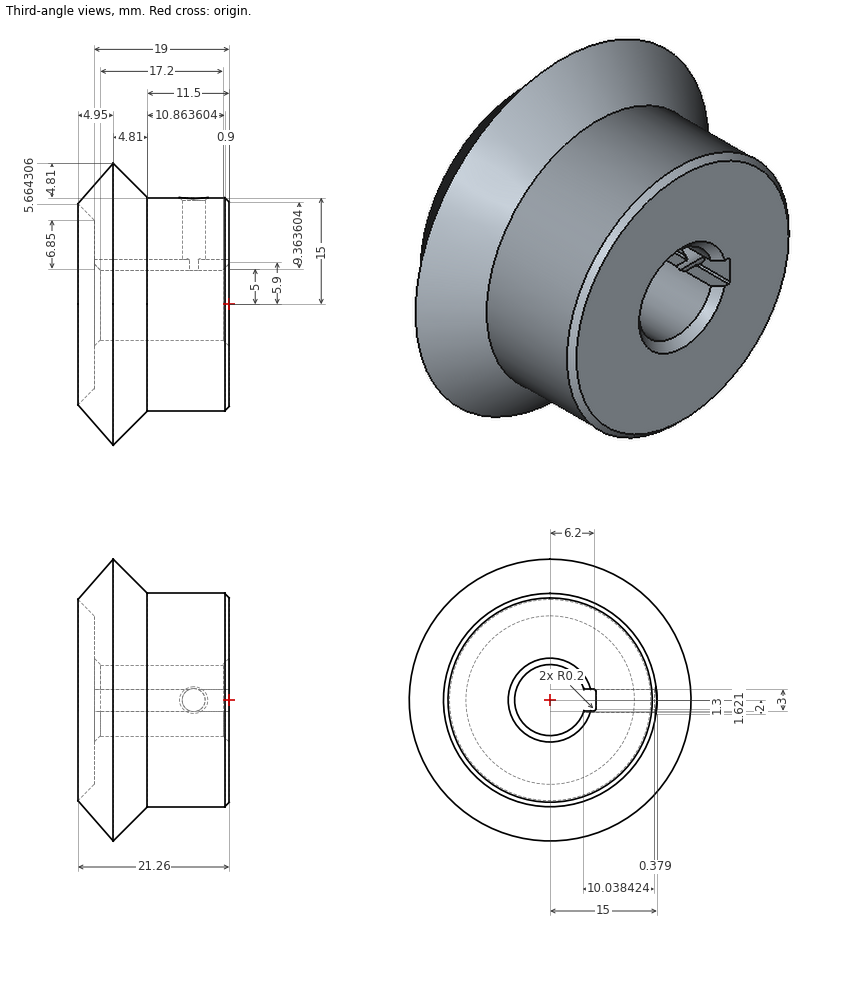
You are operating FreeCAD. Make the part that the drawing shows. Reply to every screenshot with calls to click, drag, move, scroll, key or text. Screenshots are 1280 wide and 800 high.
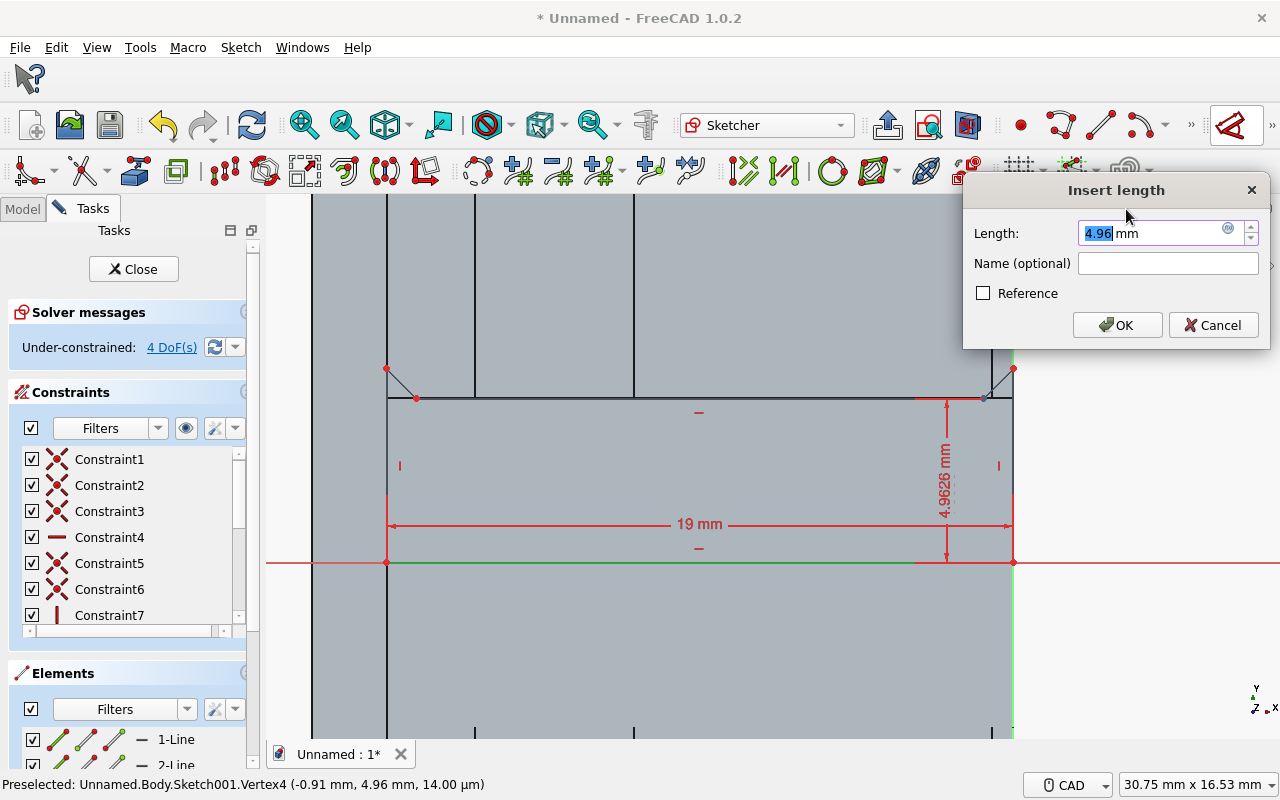
text(5)
key(Return)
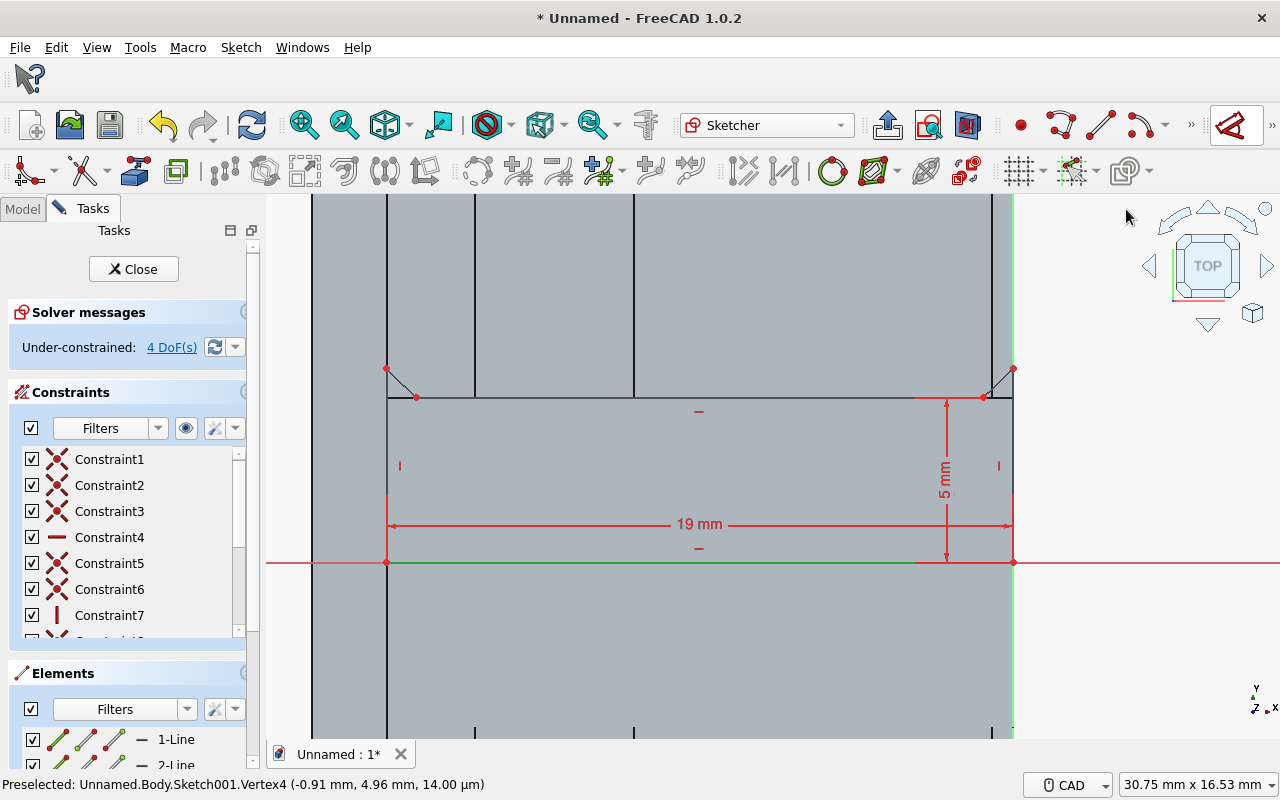
click(1013, 505)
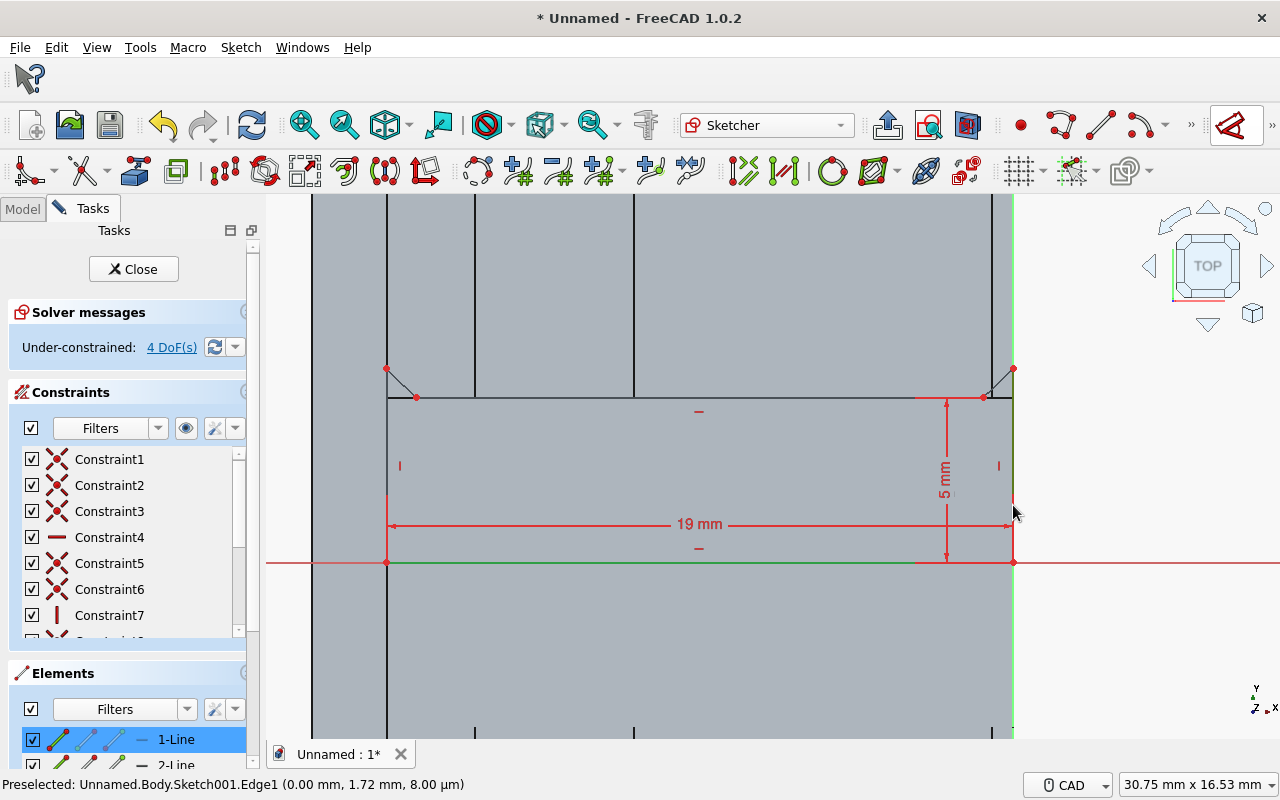
key(i)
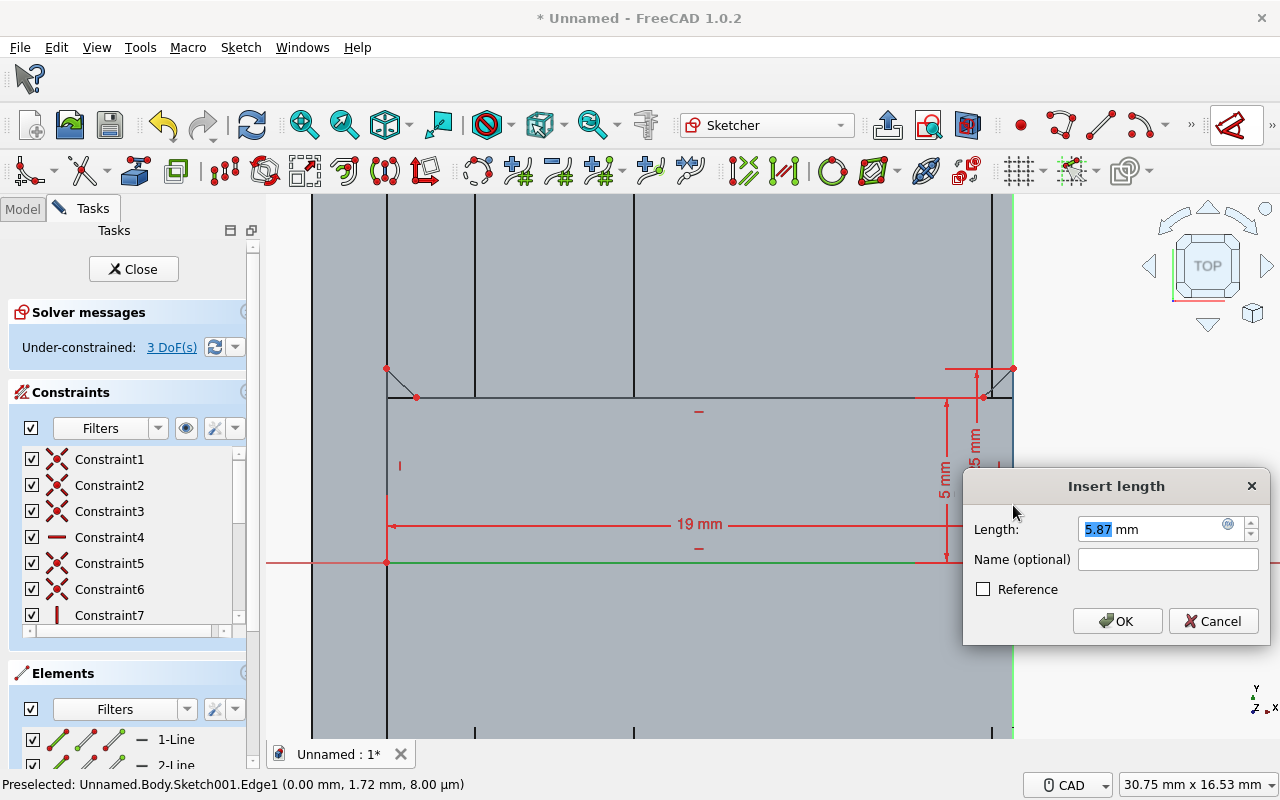
text(5.9)
key(Return)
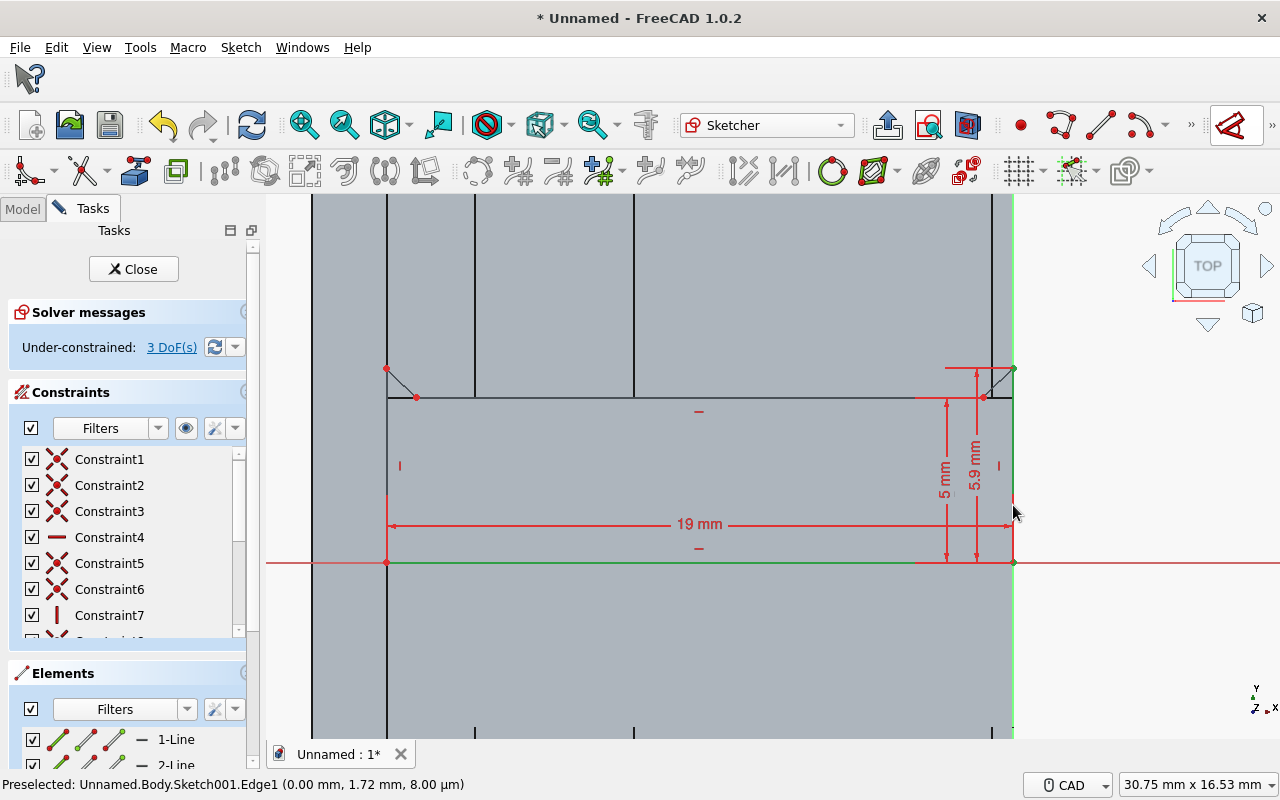
click(387, 427)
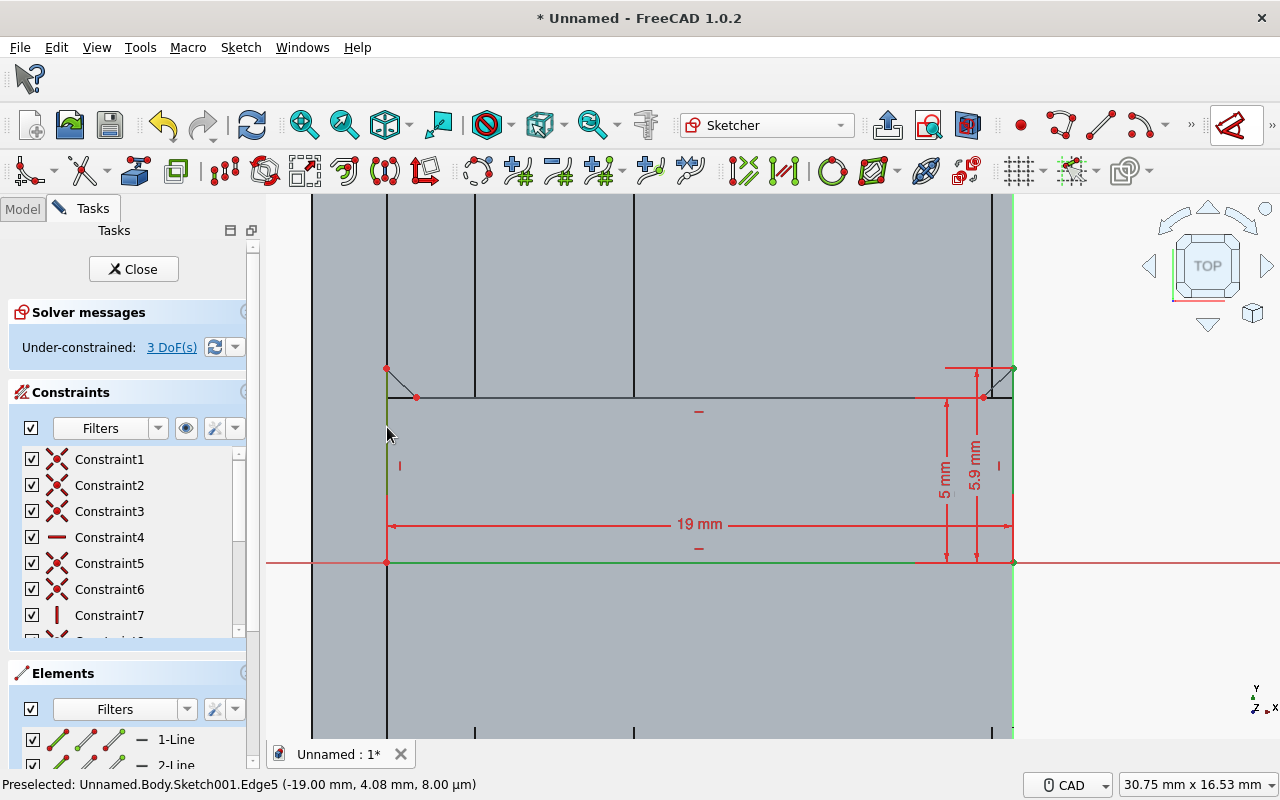
click(1258, 126)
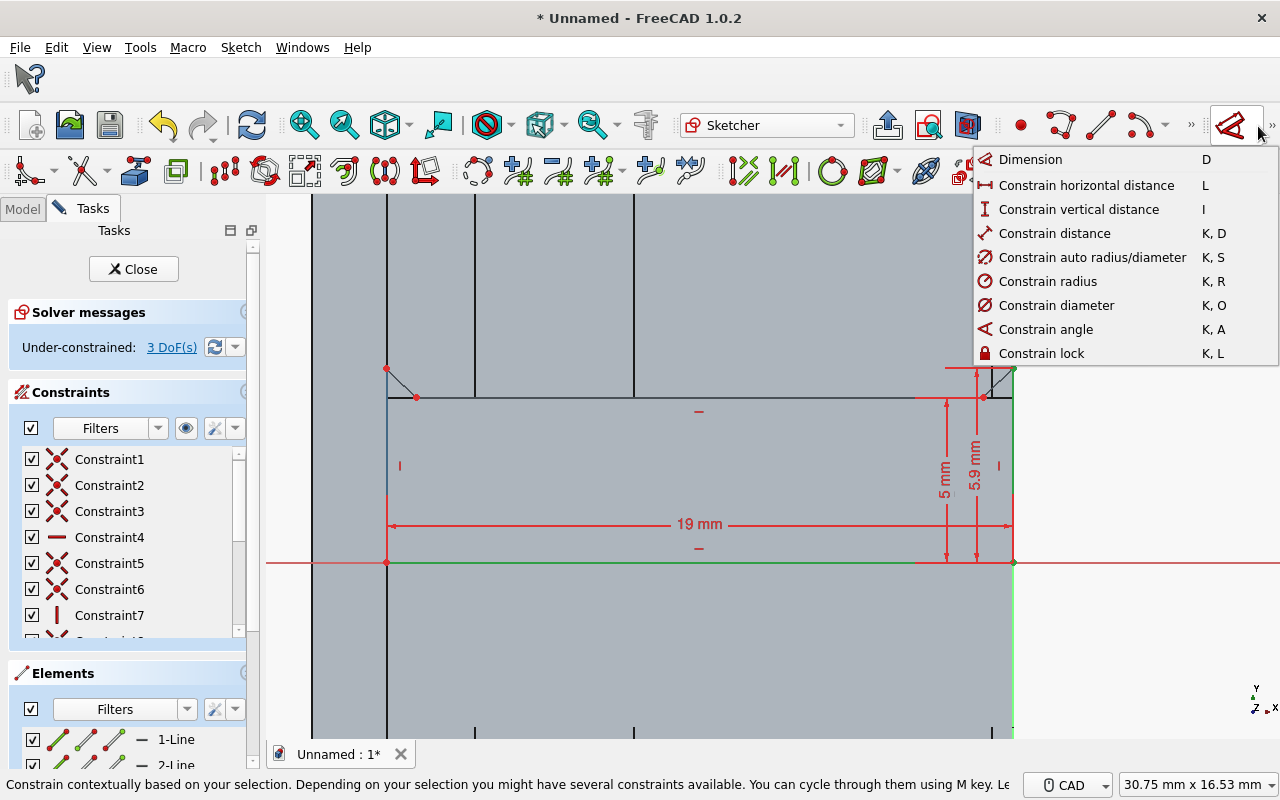
click(1126, 209)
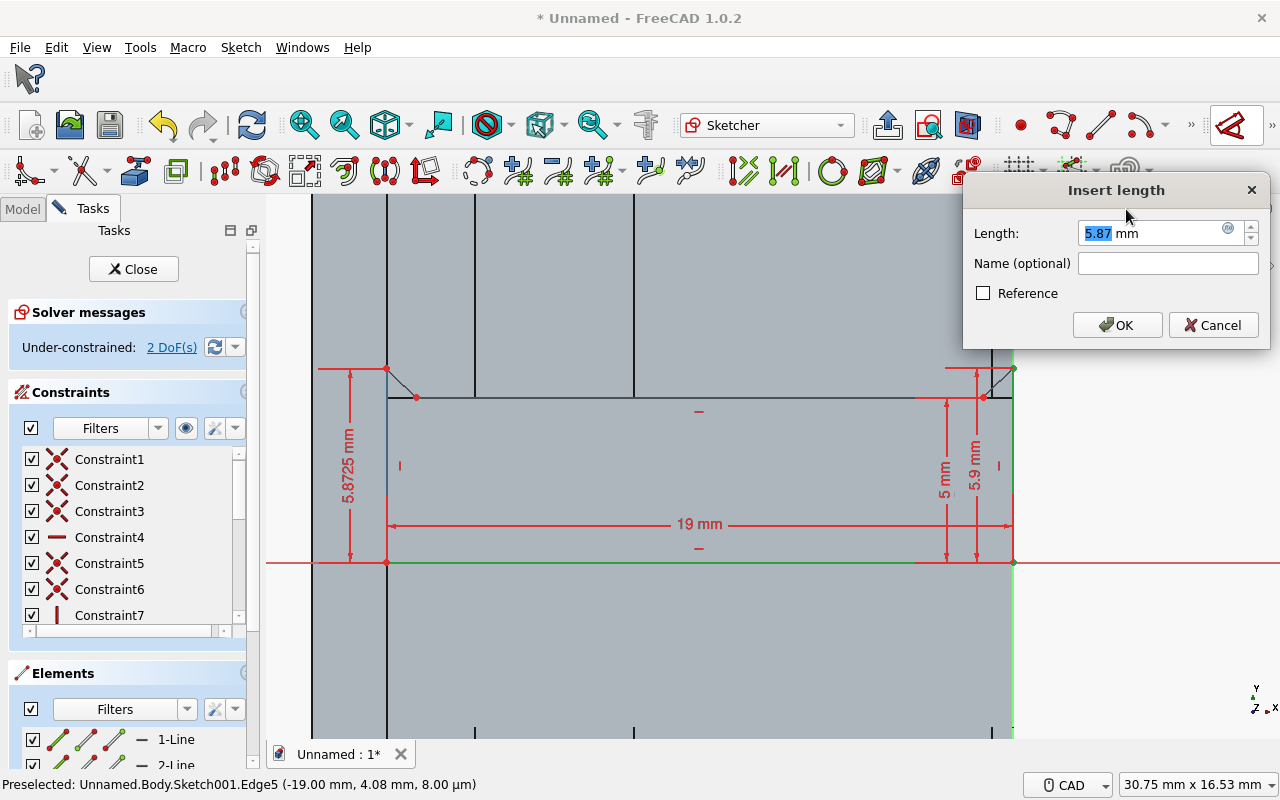
text(5.9)
key(Return)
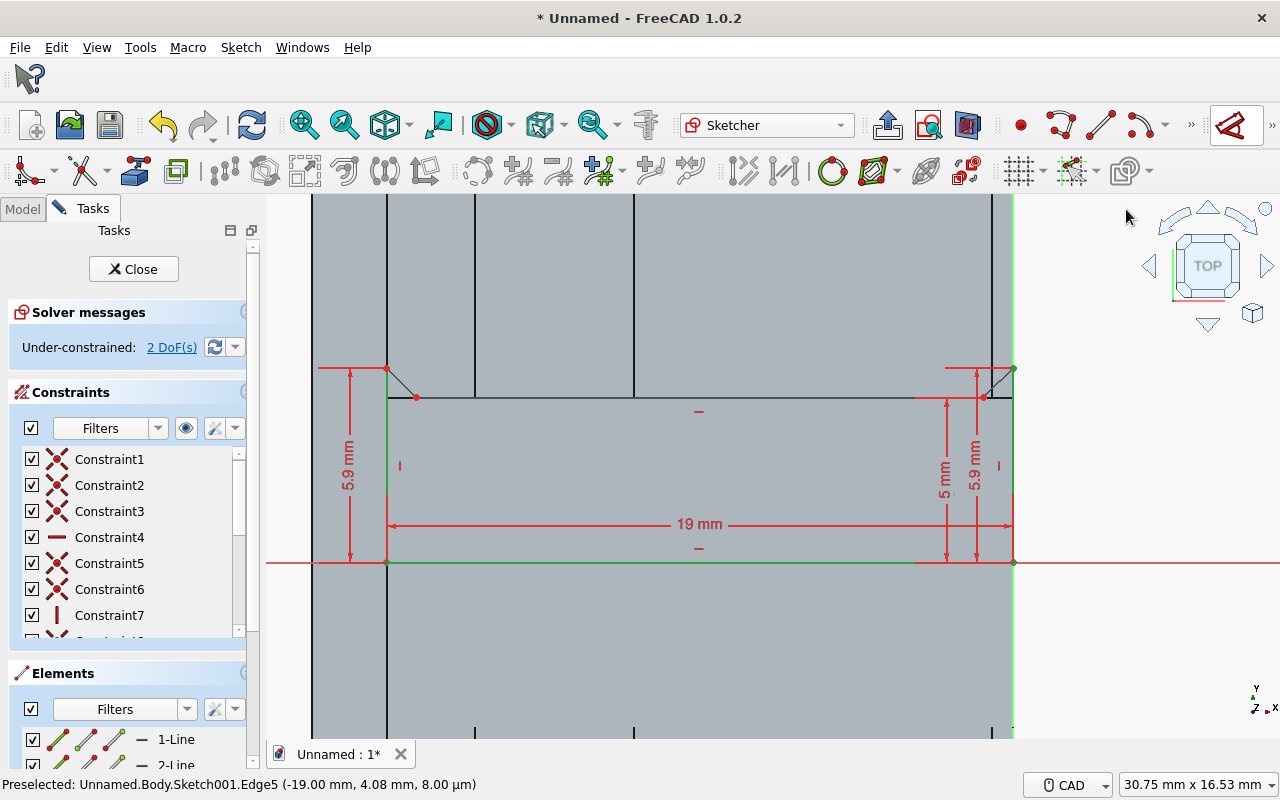
click(813, 398)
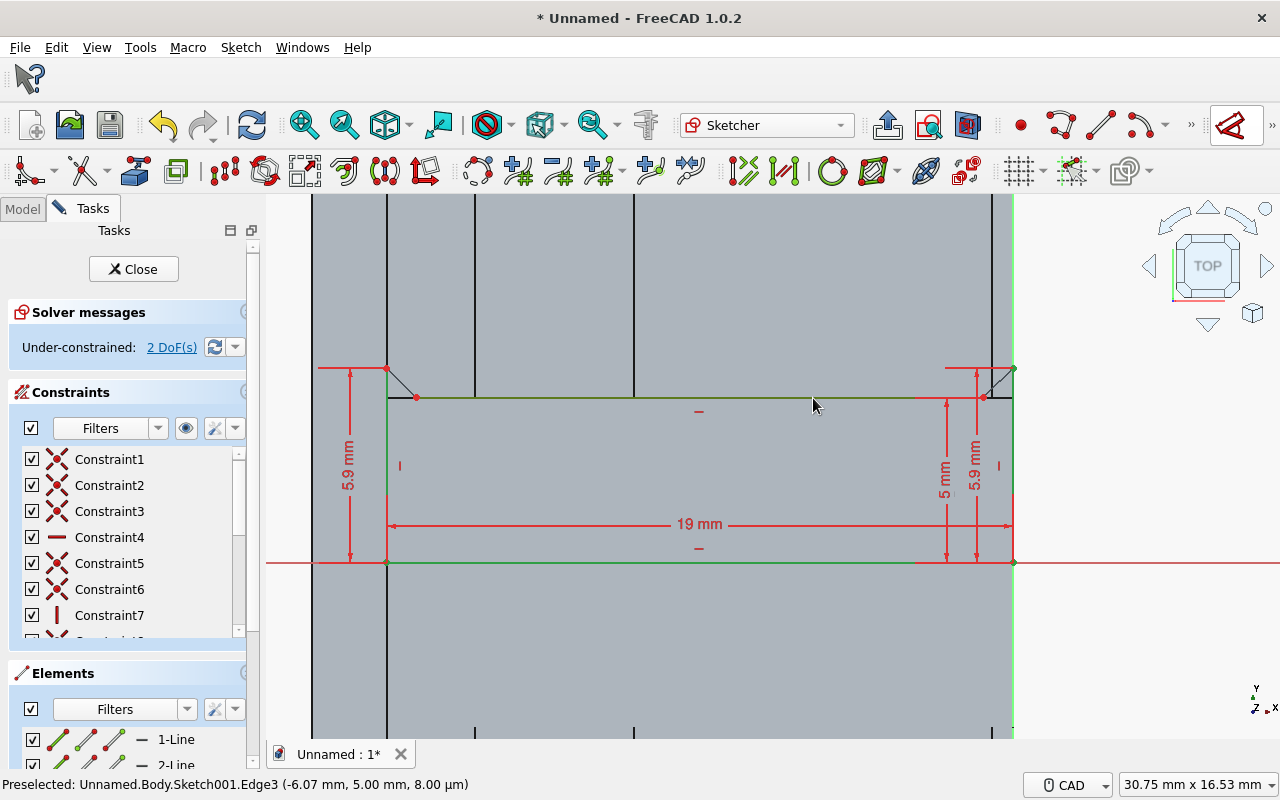
key(l)